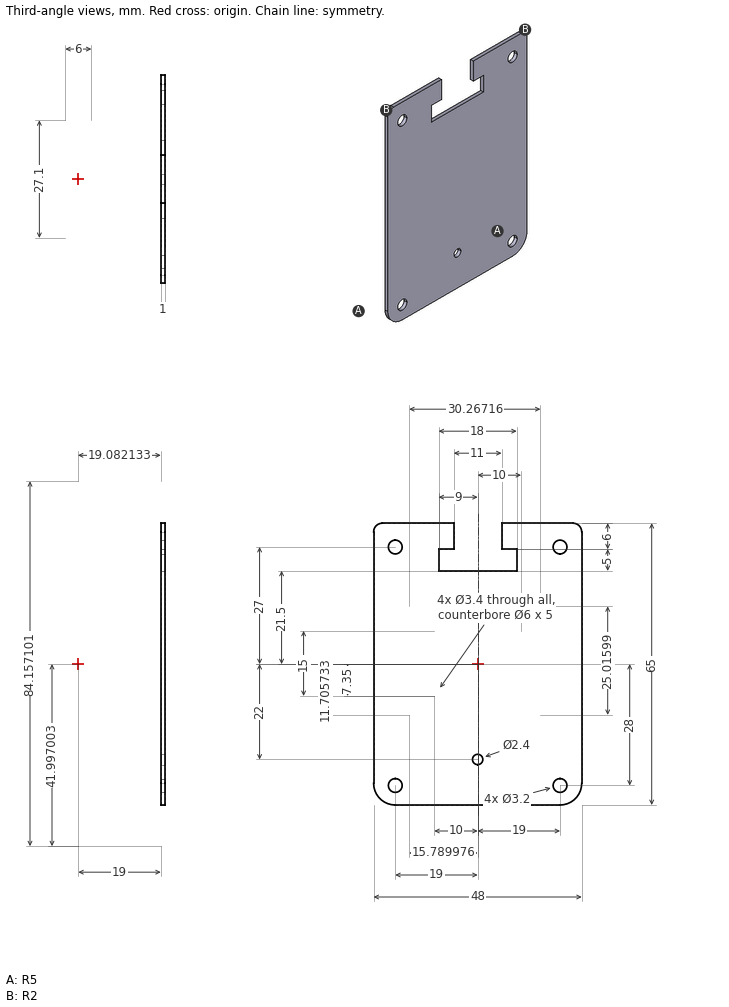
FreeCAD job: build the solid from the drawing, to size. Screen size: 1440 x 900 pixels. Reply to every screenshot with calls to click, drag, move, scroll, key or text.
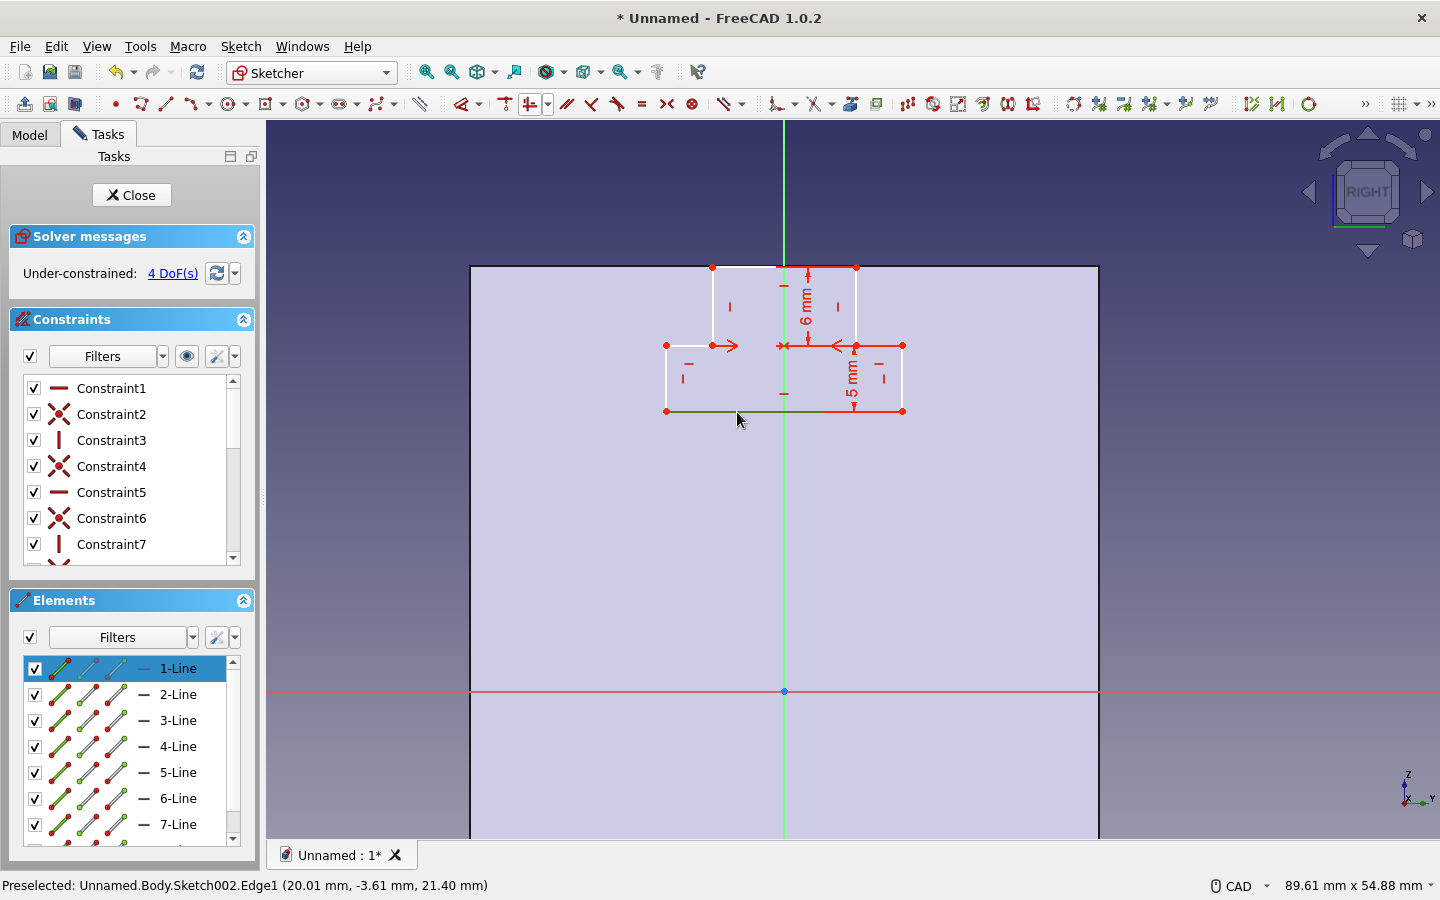
click(478, 104)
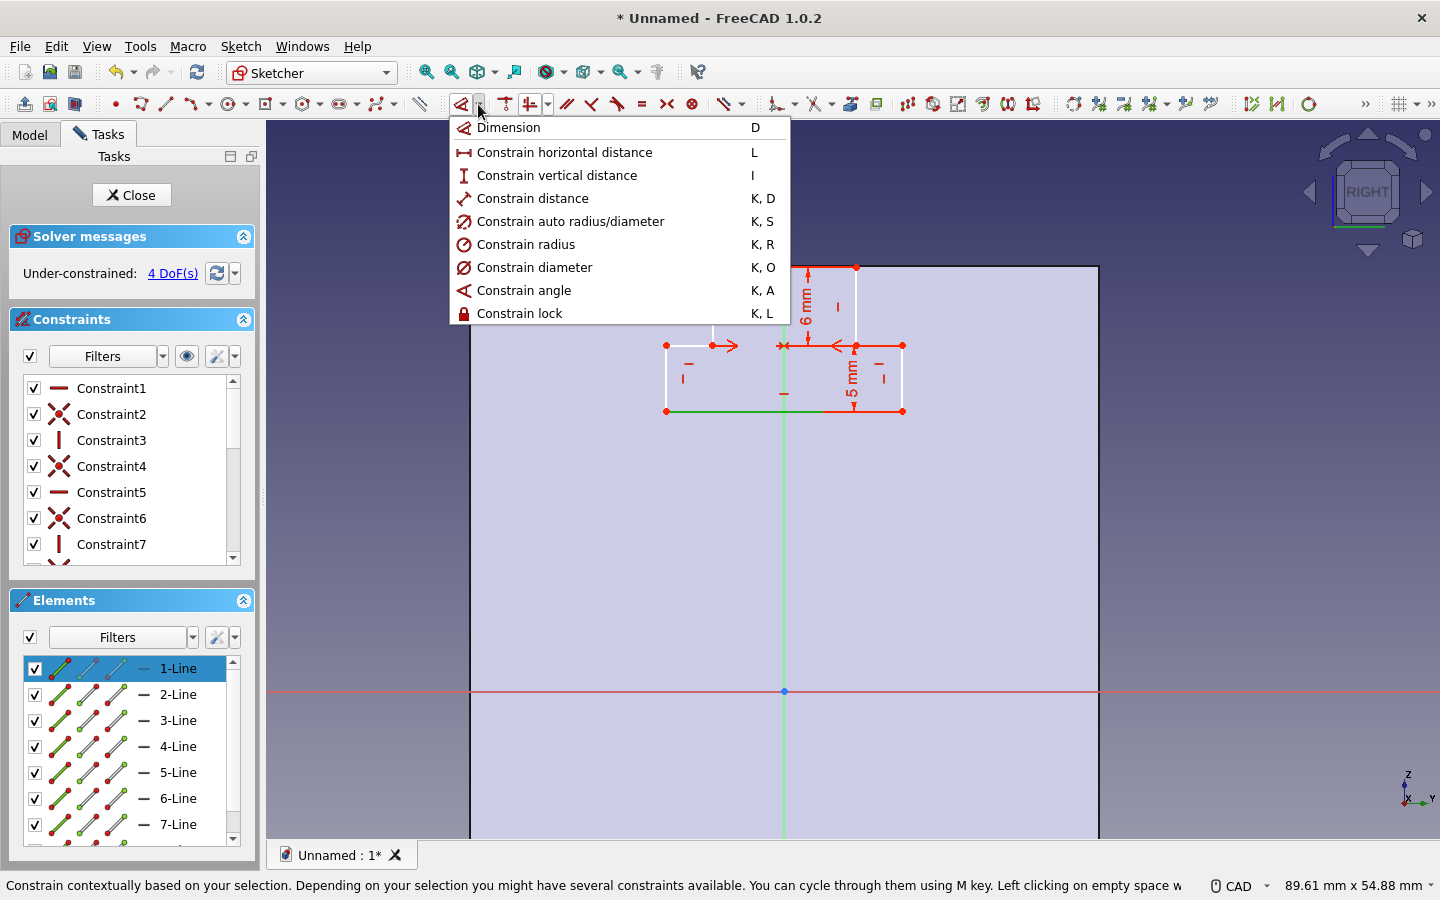
click(620, 152)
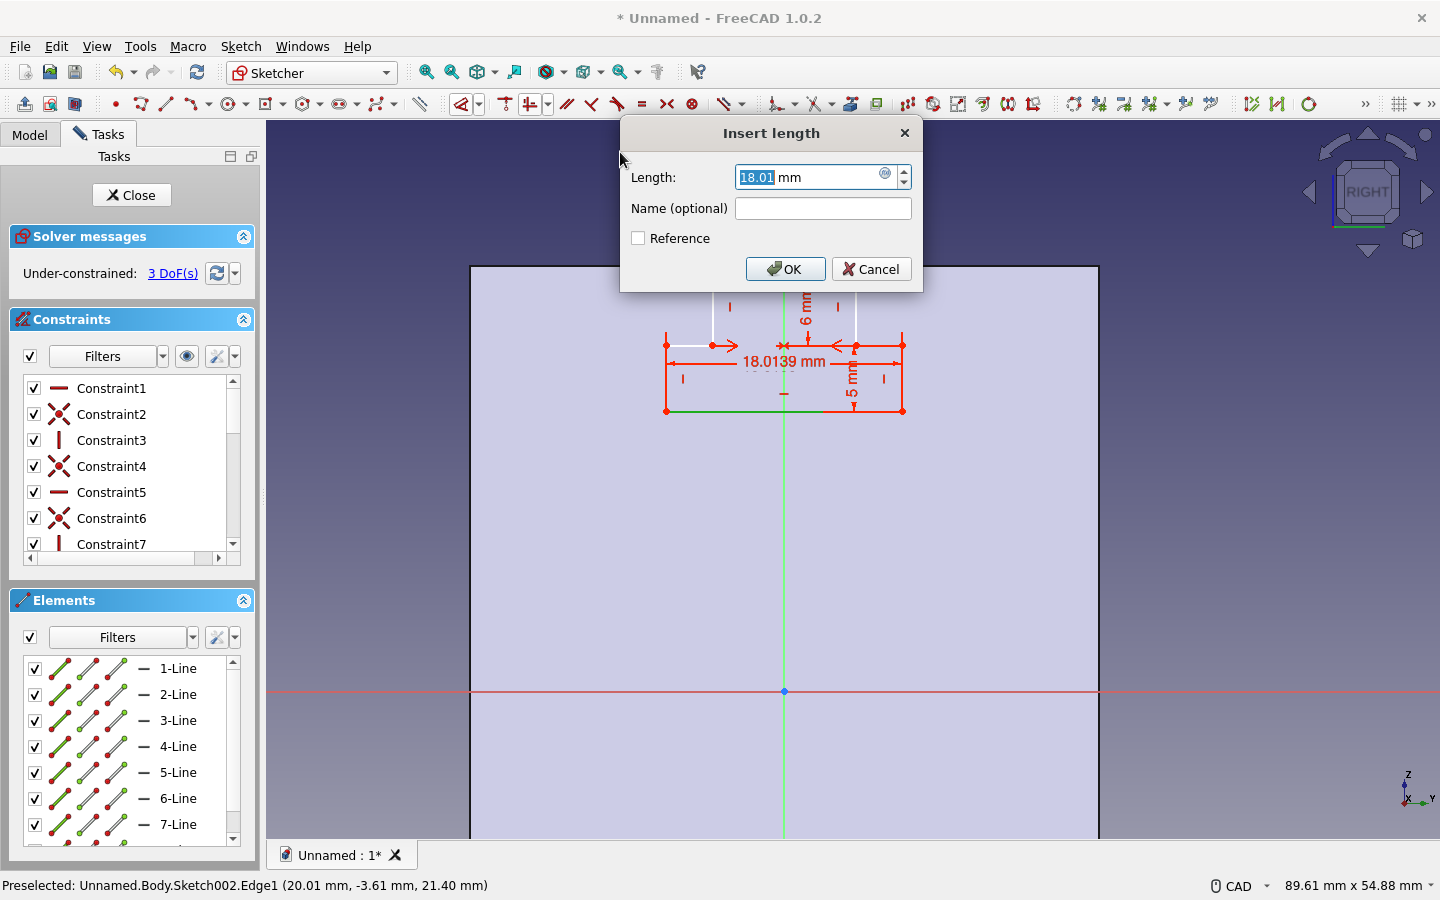
text(18)
key(Return)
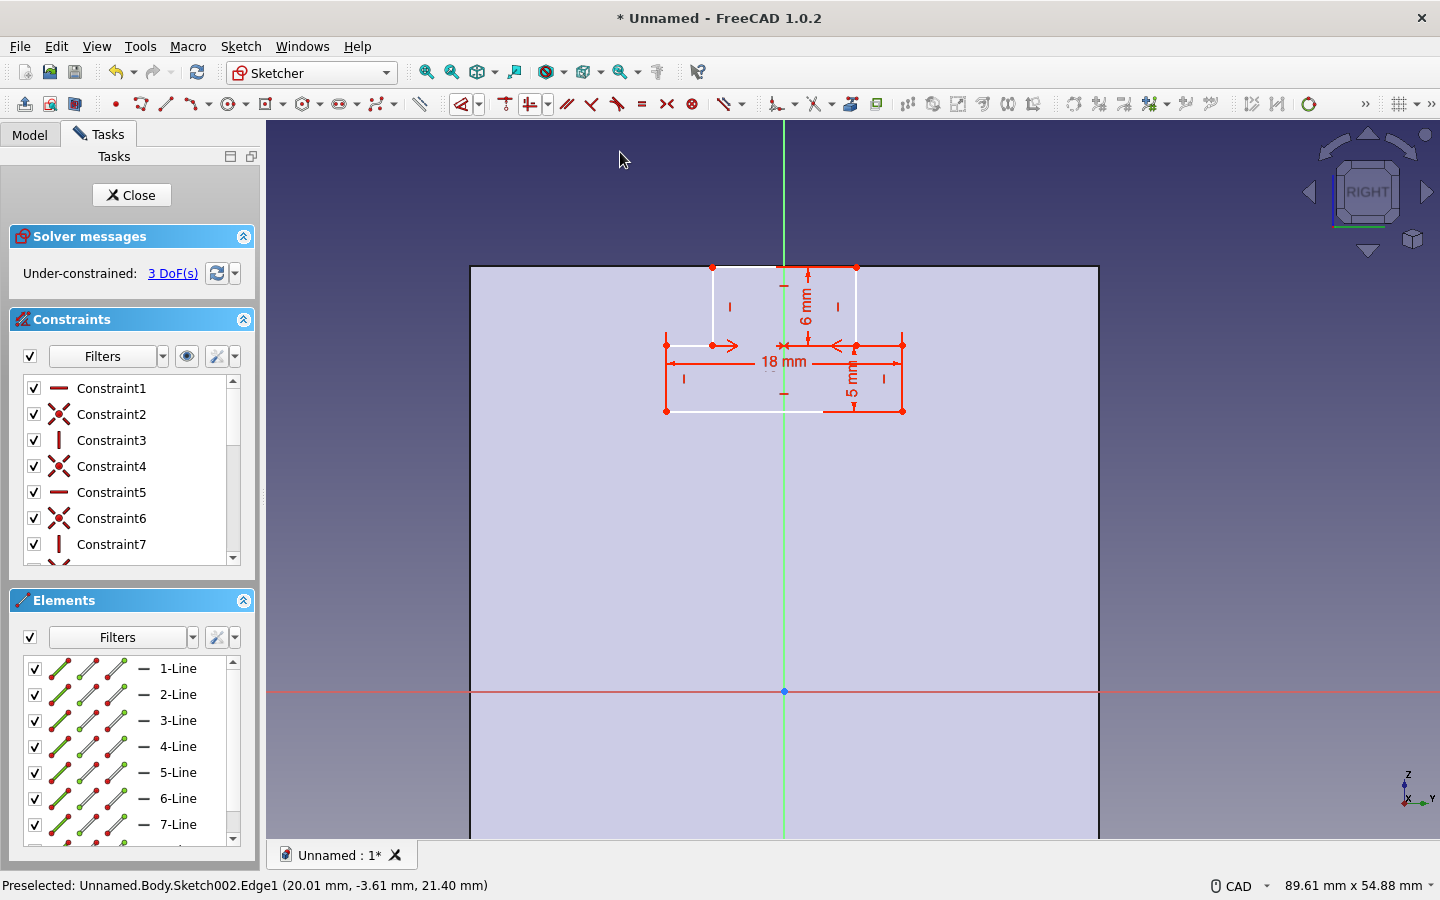
click(813, 267)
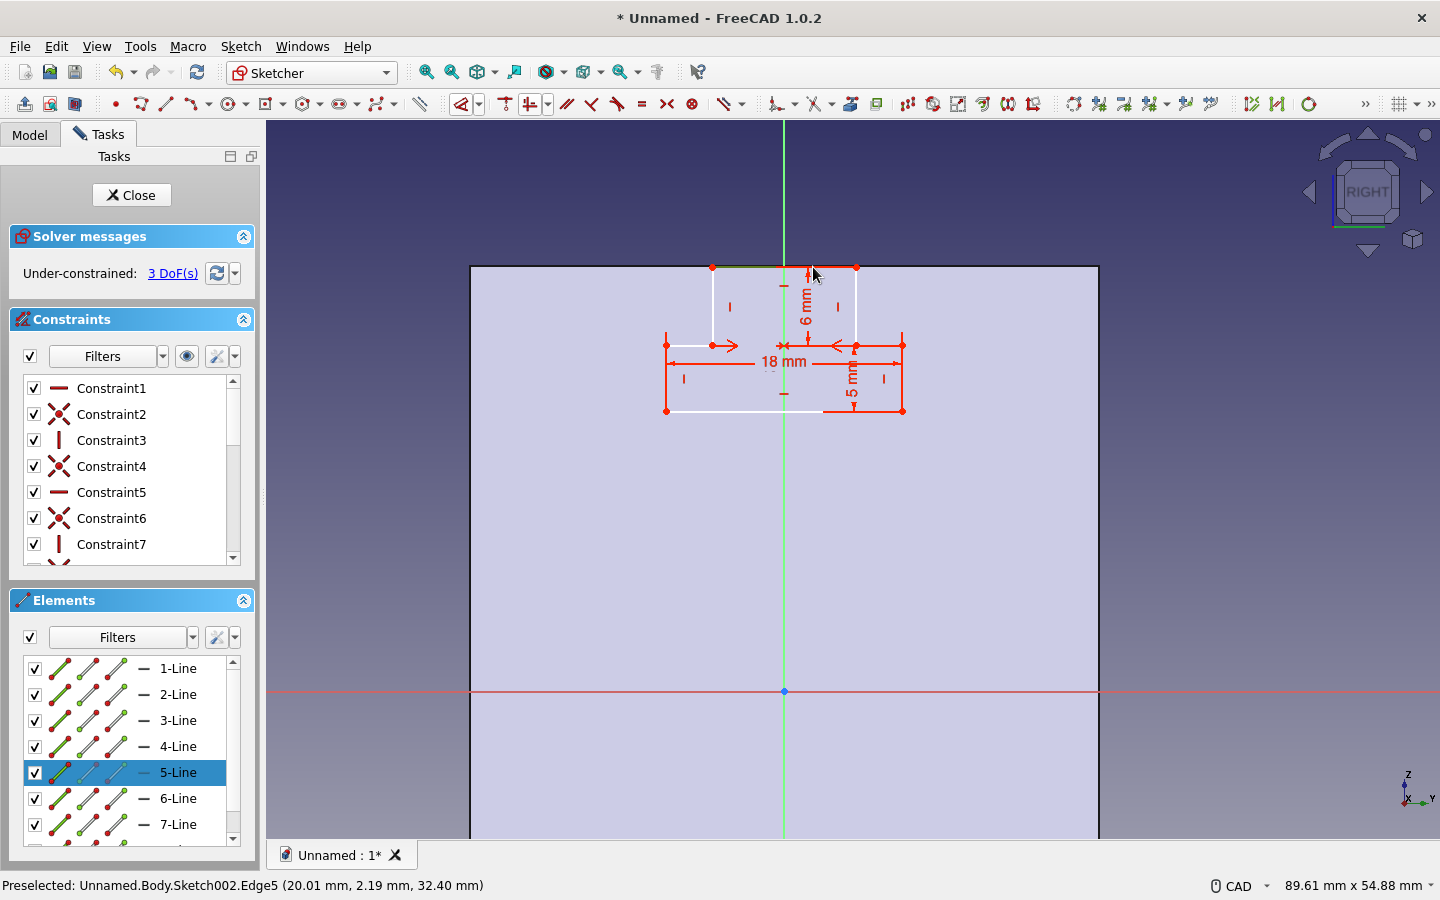
key(l)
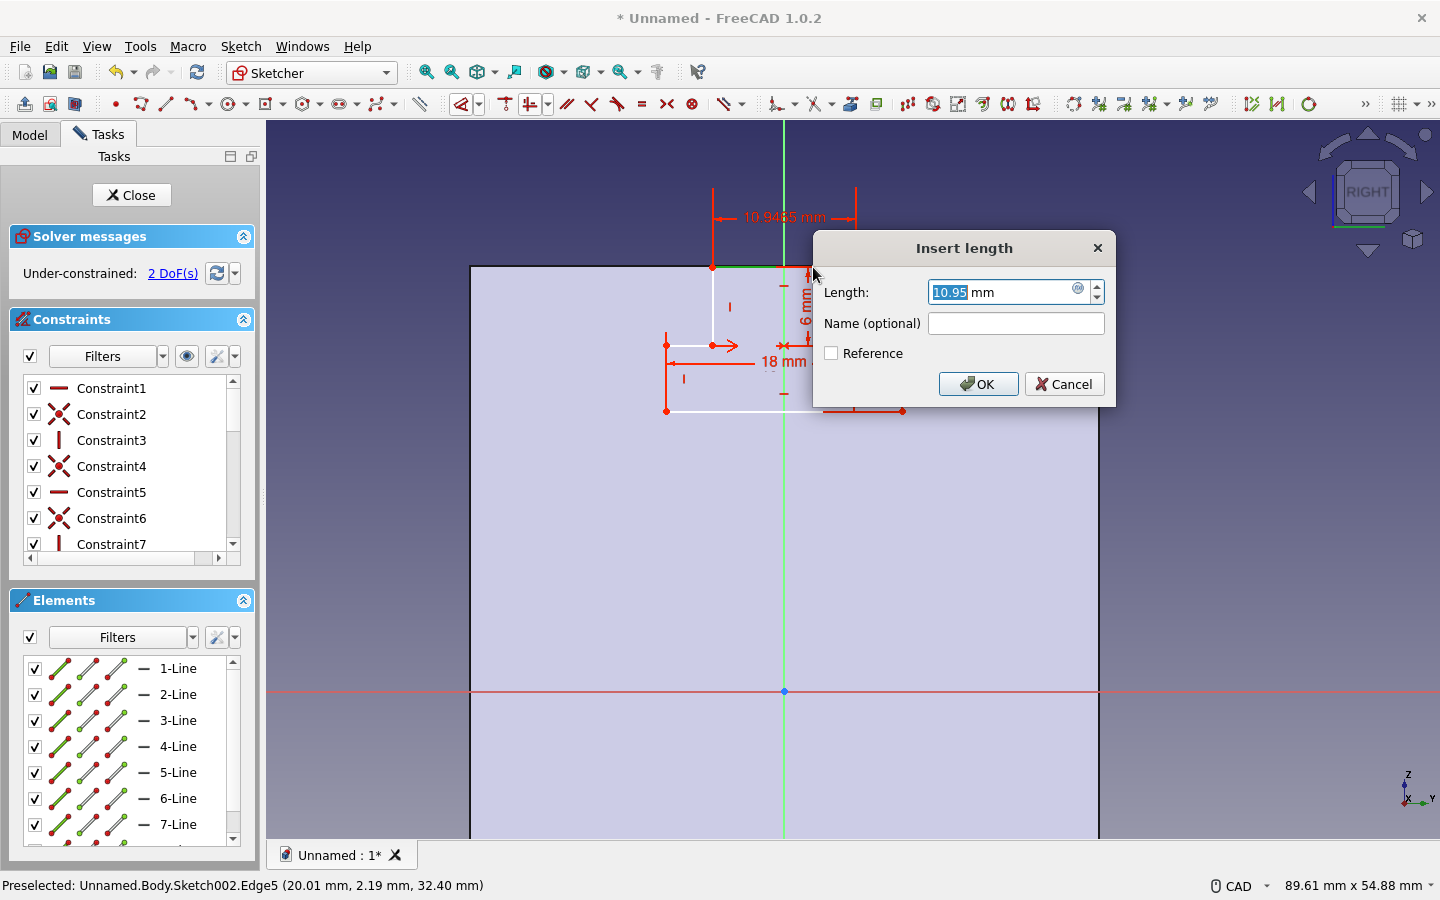
text(11)
key(Return)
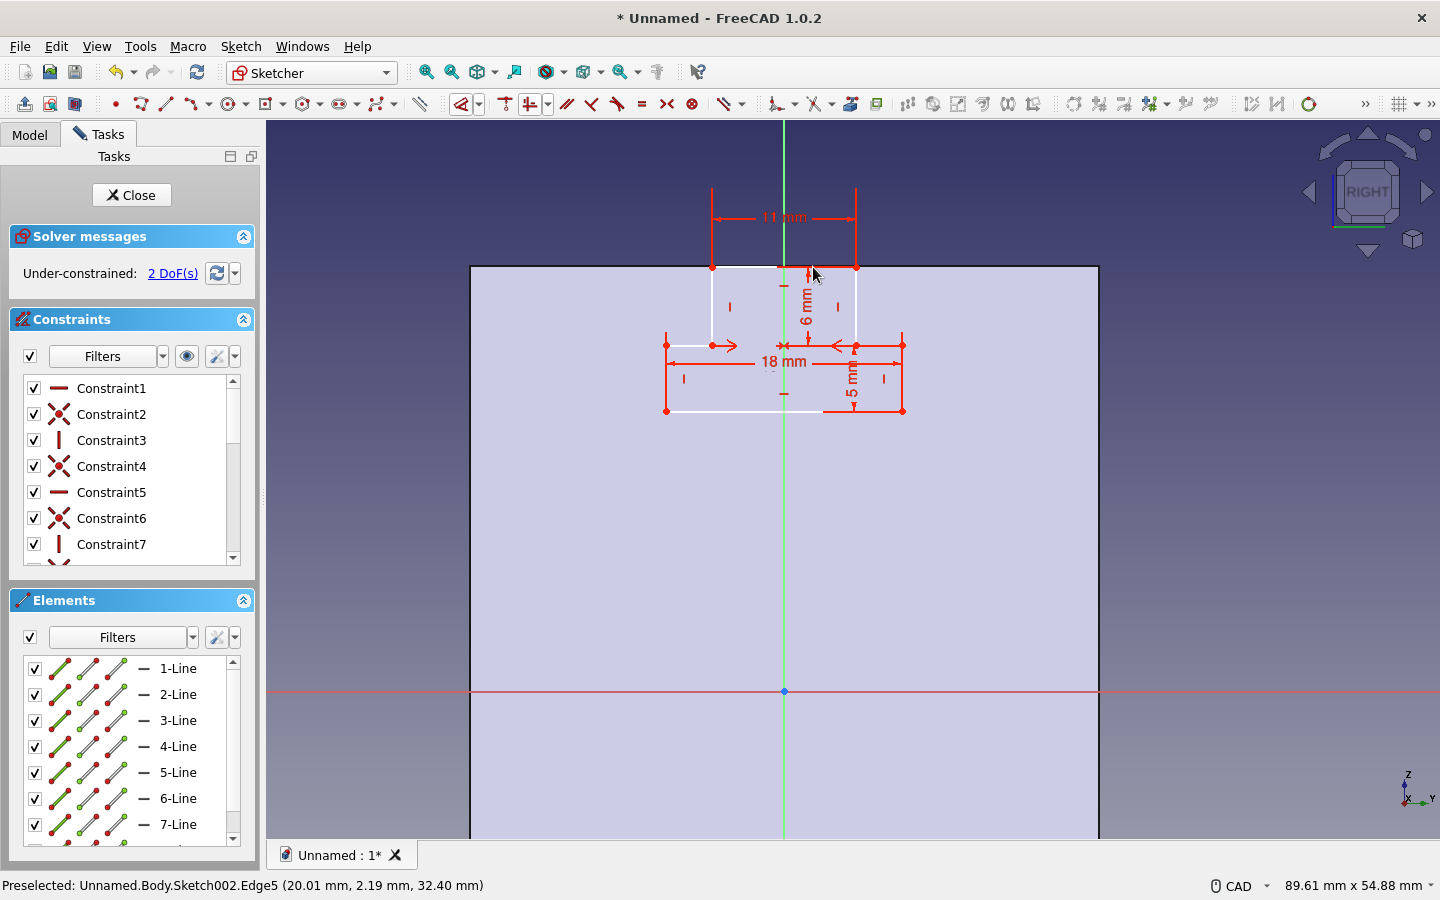
click(666, 412)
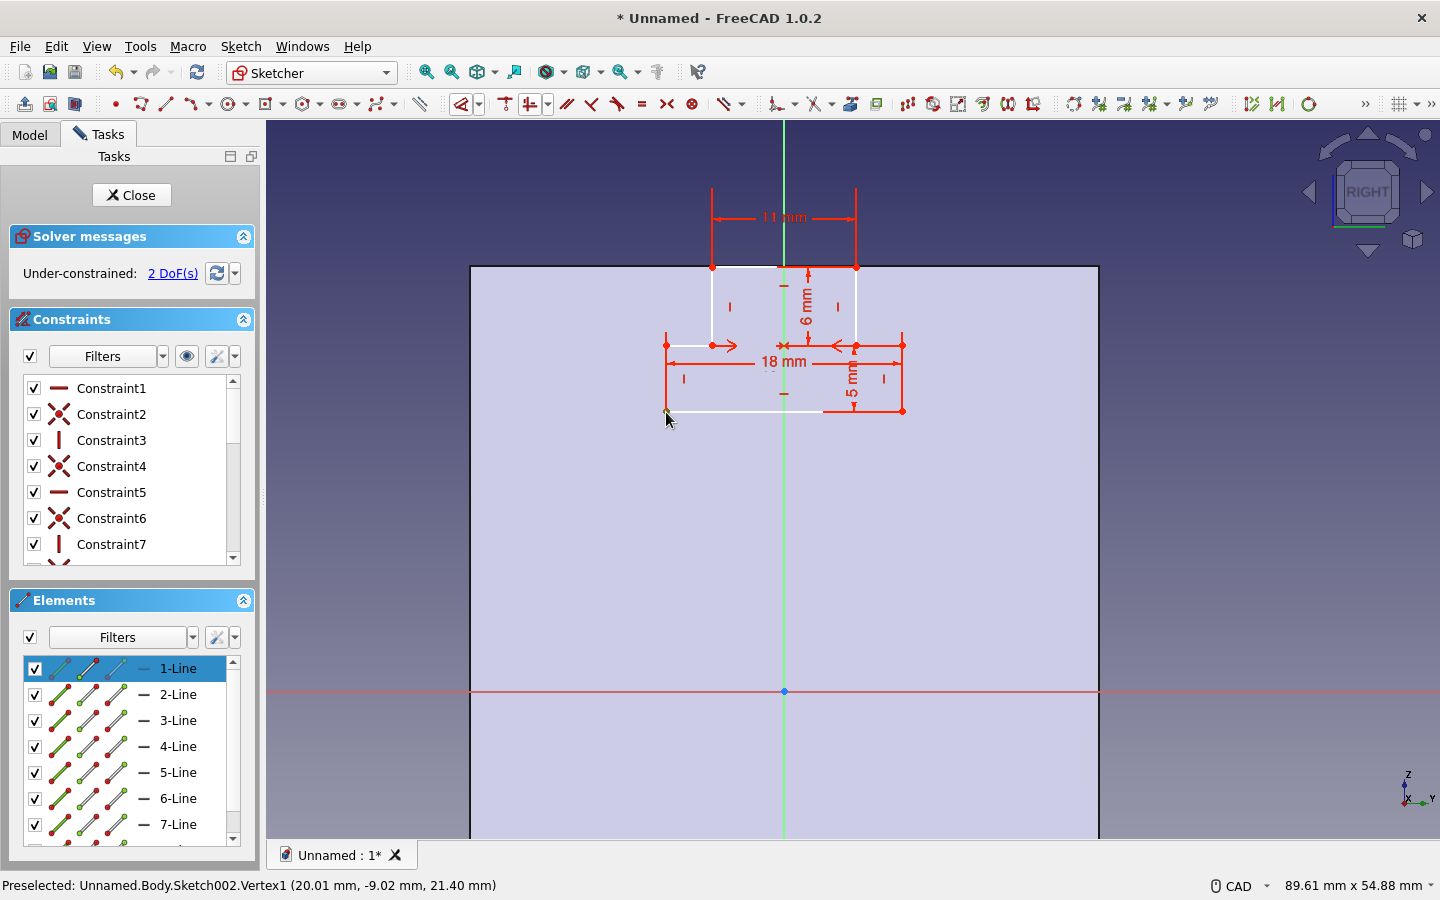
key(l)